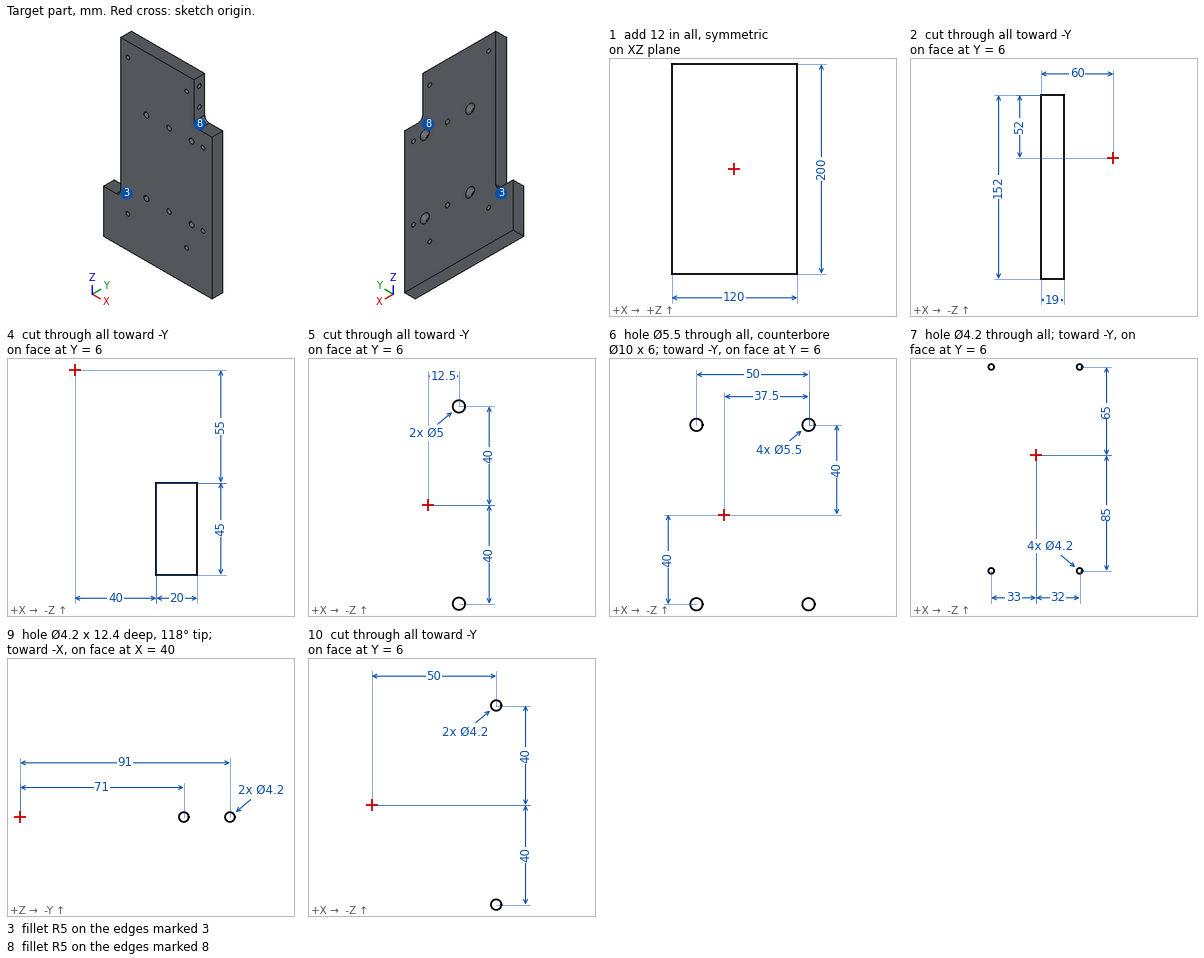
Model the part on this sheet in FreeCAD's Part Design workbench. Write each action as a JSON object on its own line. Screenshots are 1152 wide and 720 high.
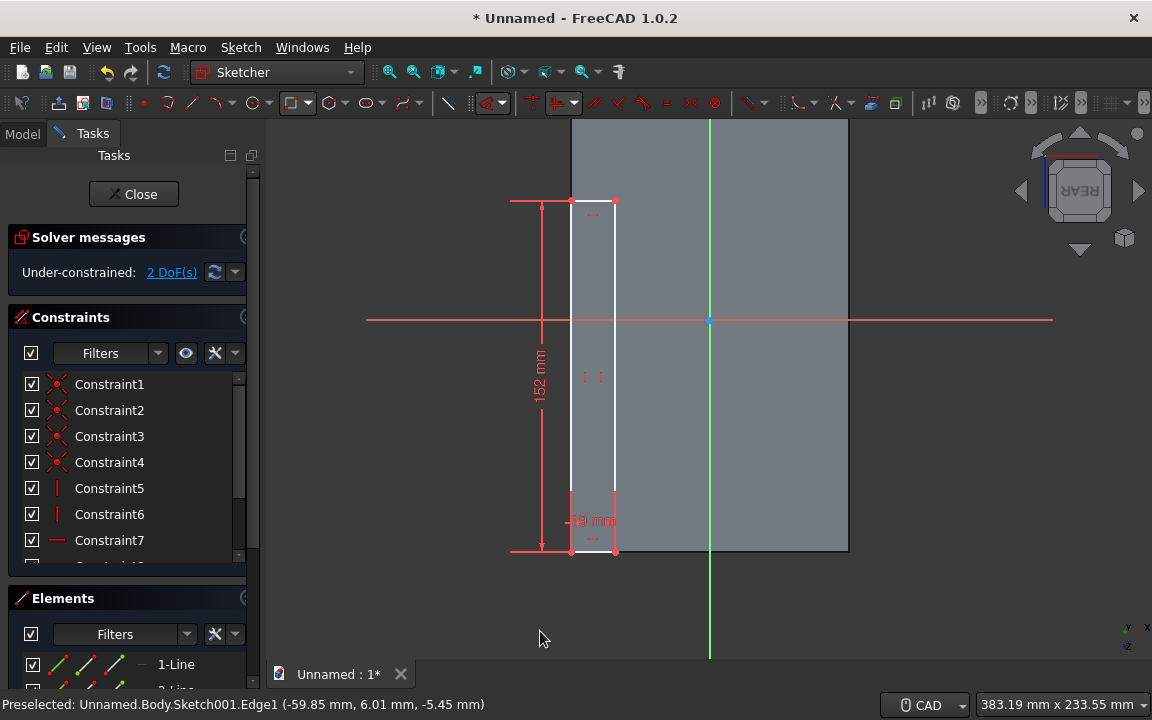
{"action": "left_click", "coordinate": [572, 201]}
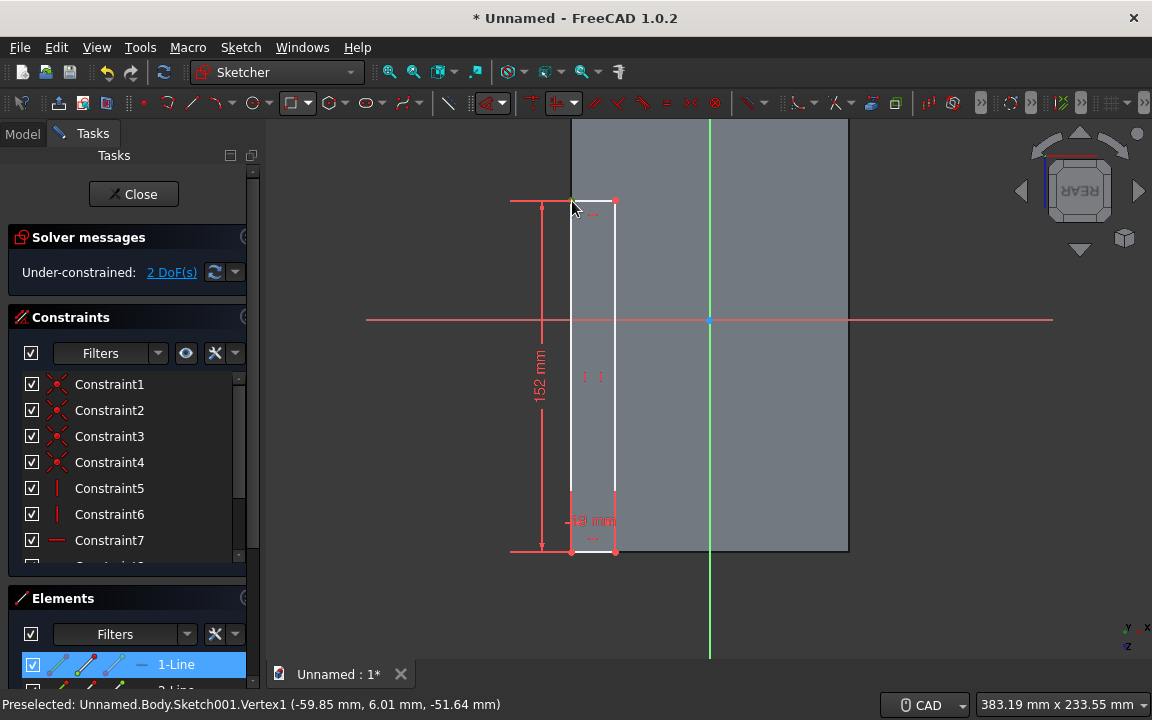
{"action": "key", "text": "l"}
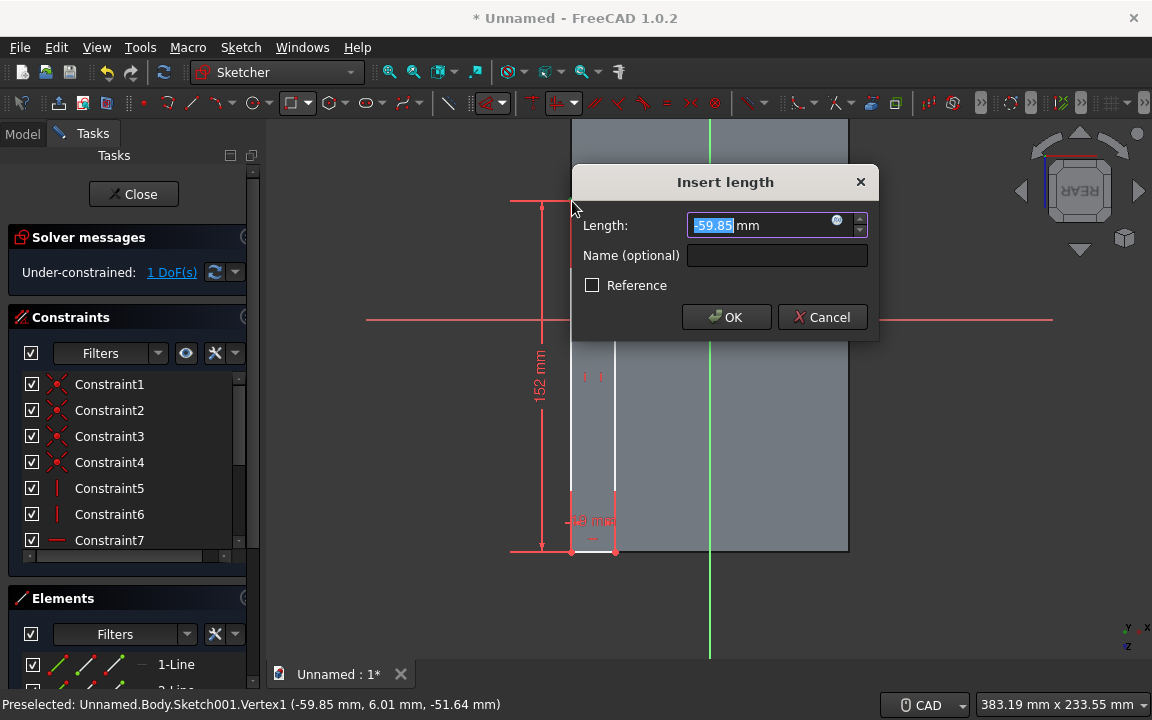
{"action": "type", "text": "-60"}
{"action": "key", "text": "Return"}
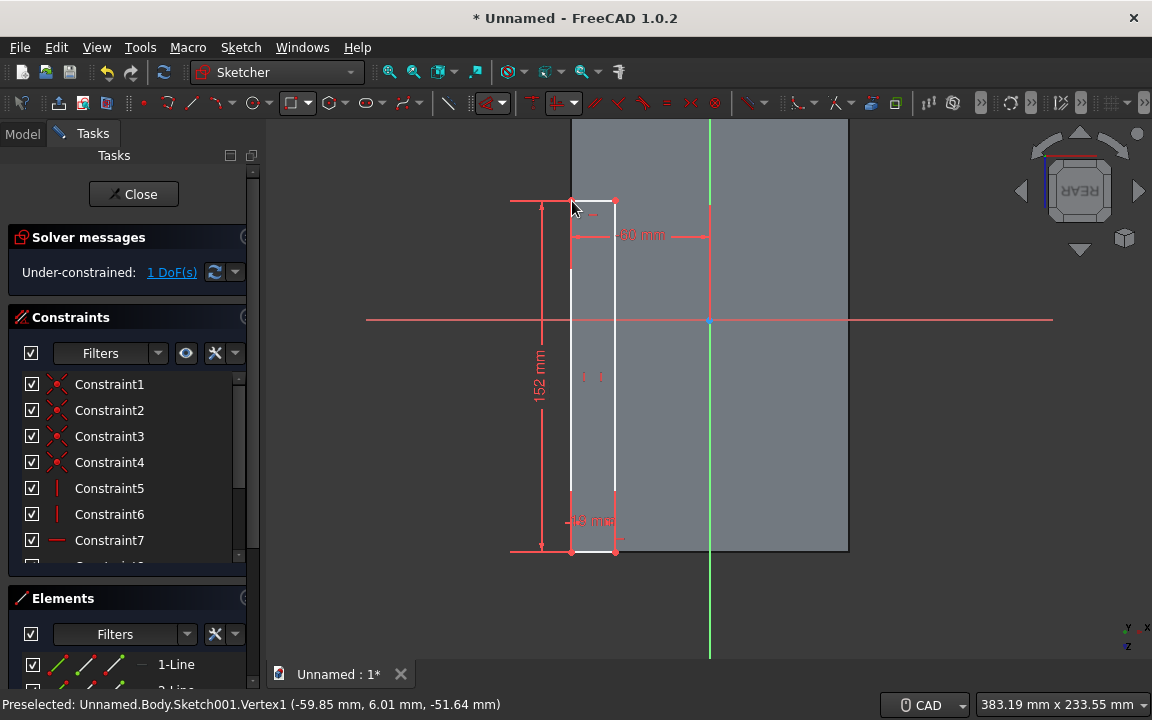
{"action": "left_click", "coordinate": [571, 201]}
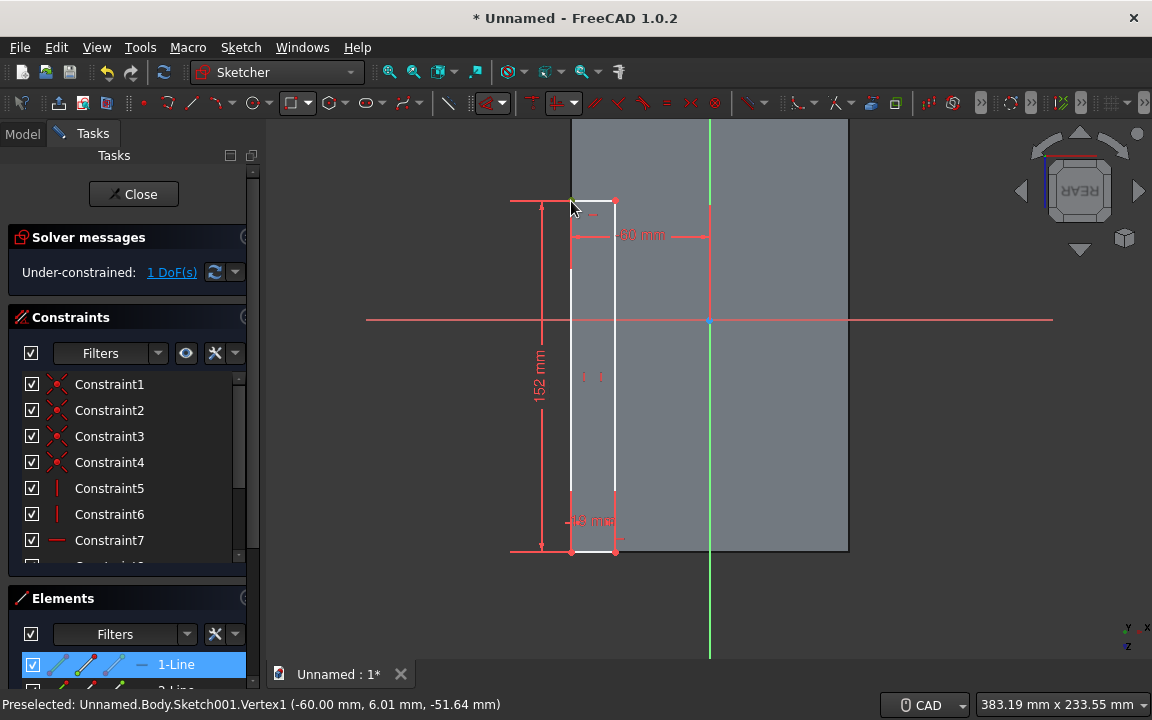
{"action": "left_click", "coordinate": [504, 104]}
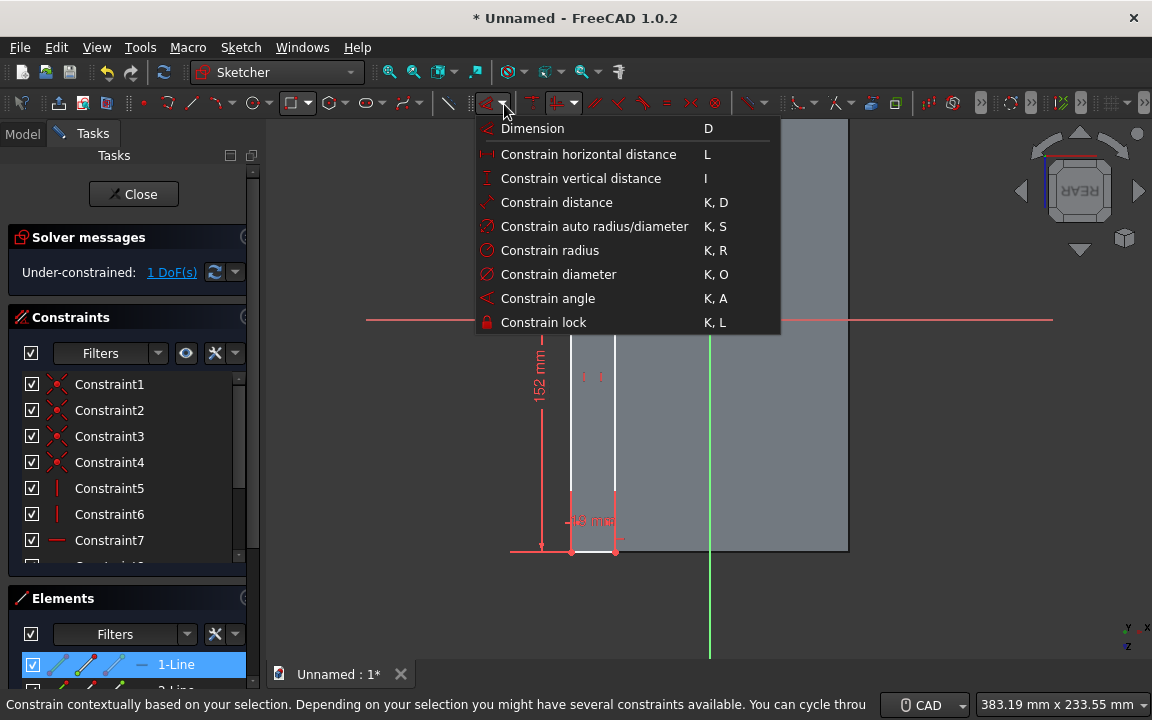
{"action": "left_click", "coordinate": [628, 178]}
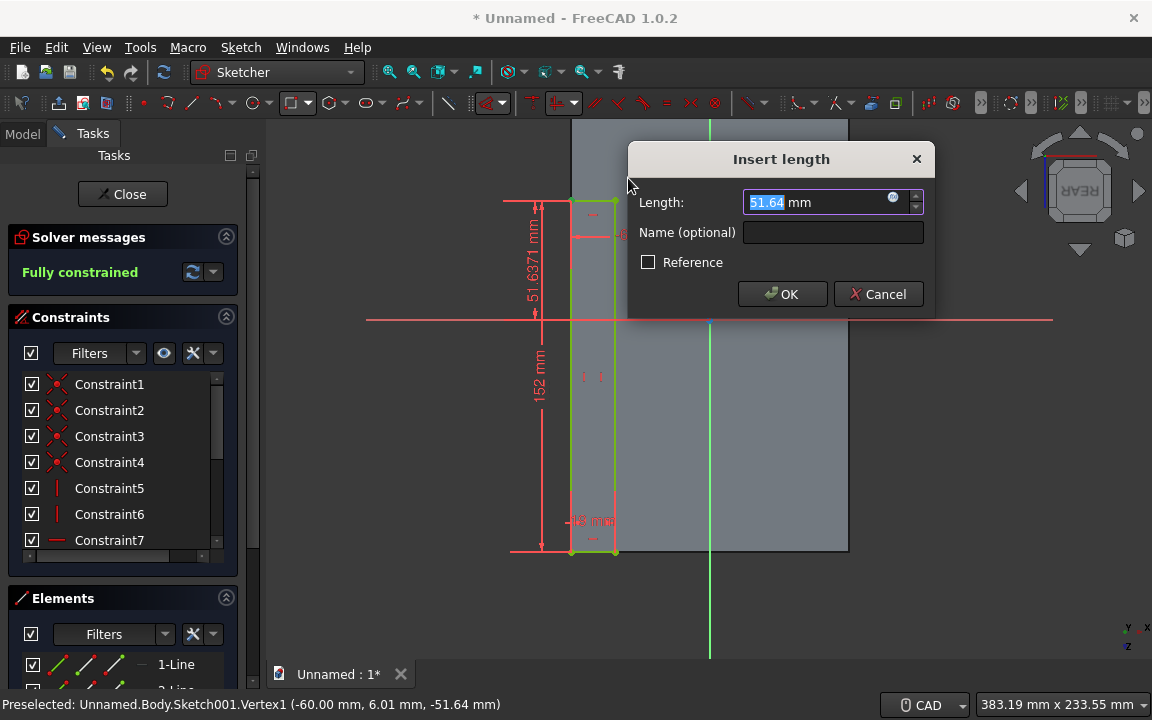
{"action": "type", "text": "52"}
{"action": "key", "text": "Return"}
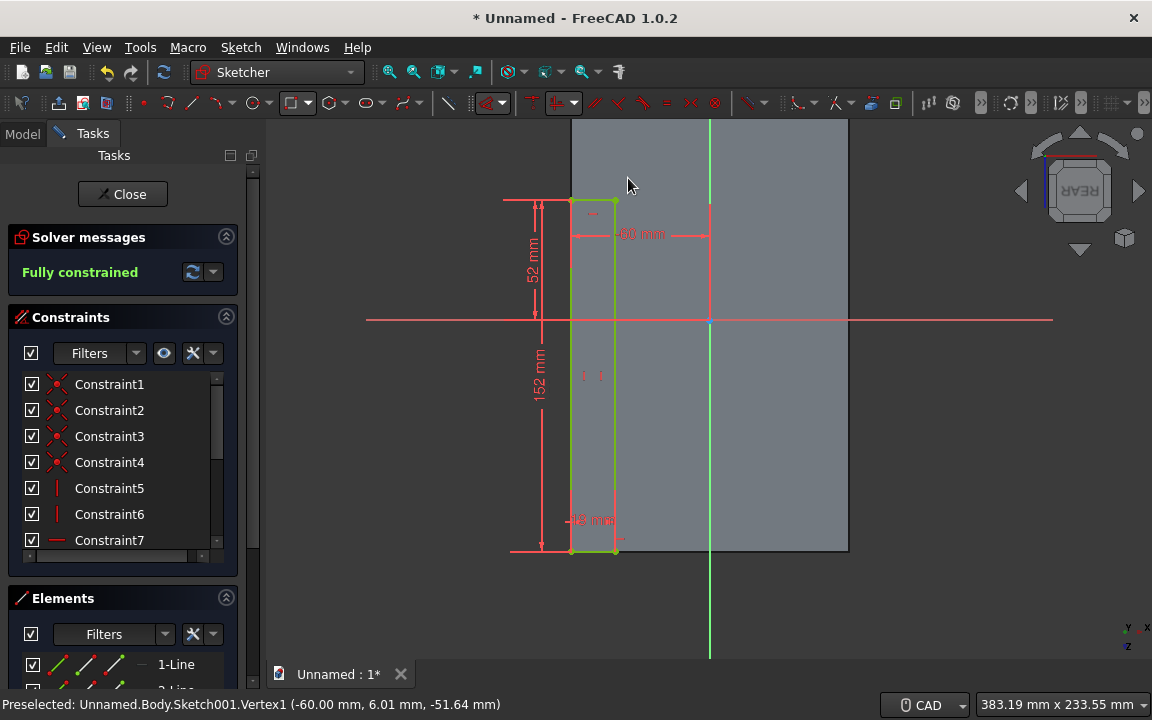
{"action": "left_click", "coordinate": [123, 194]}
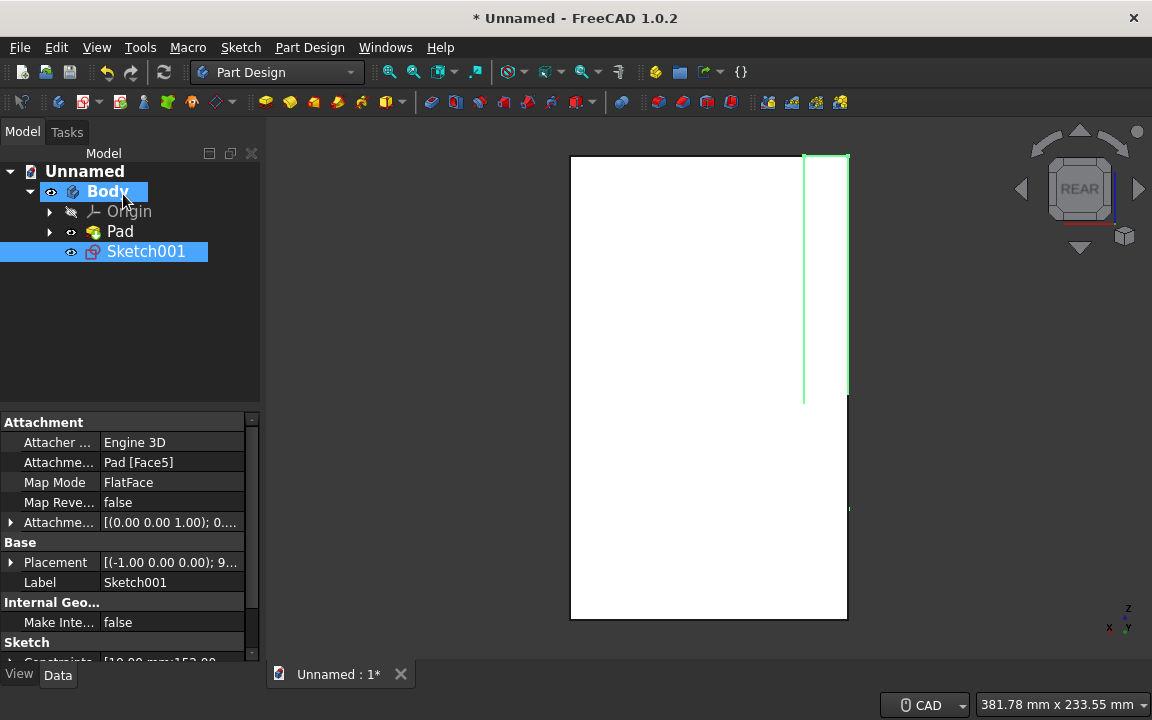
{"action": "left_click", "coordinate": [432, 102]}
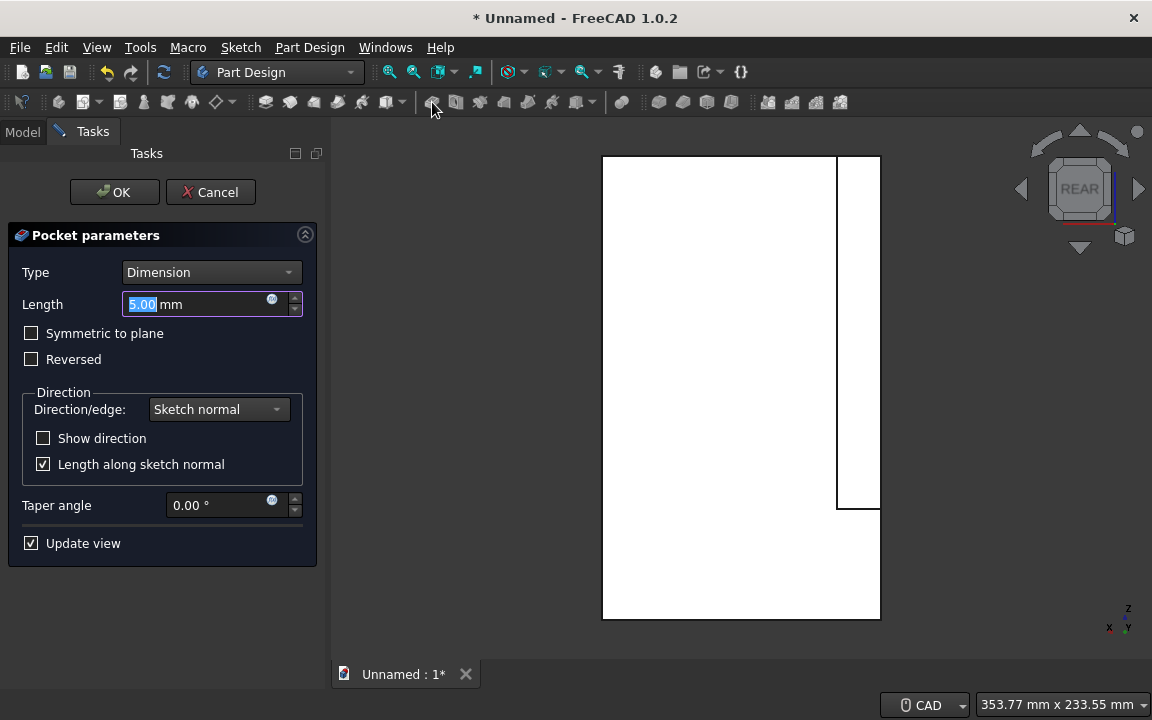
{"action": "left_click", "coordinate": [212, 272]}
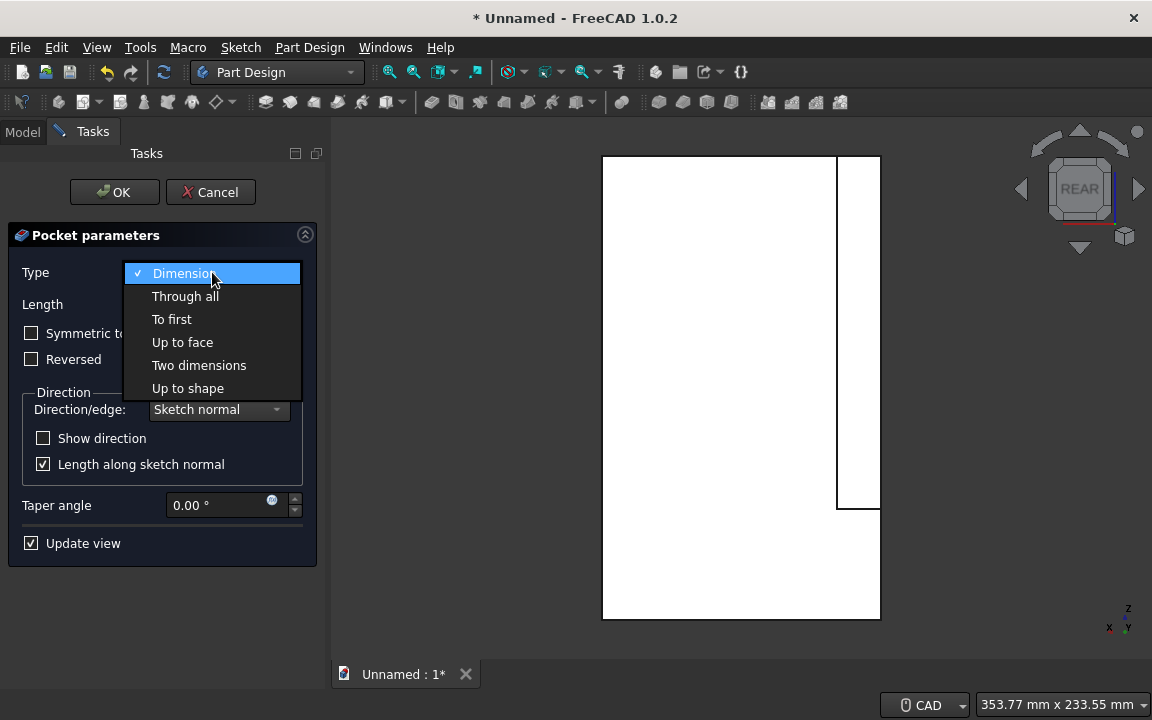
{"action": "left_click", "coordinate": [212, 296]}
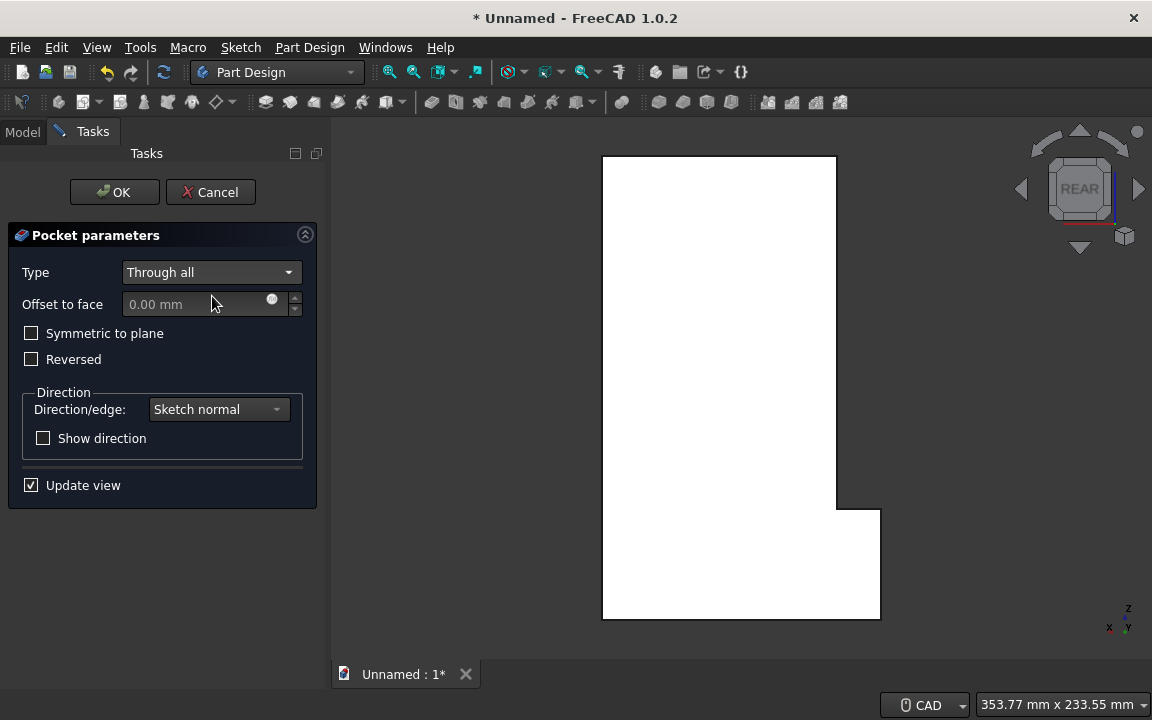
{"action": "left_click", "coordinate": [115, 192]}